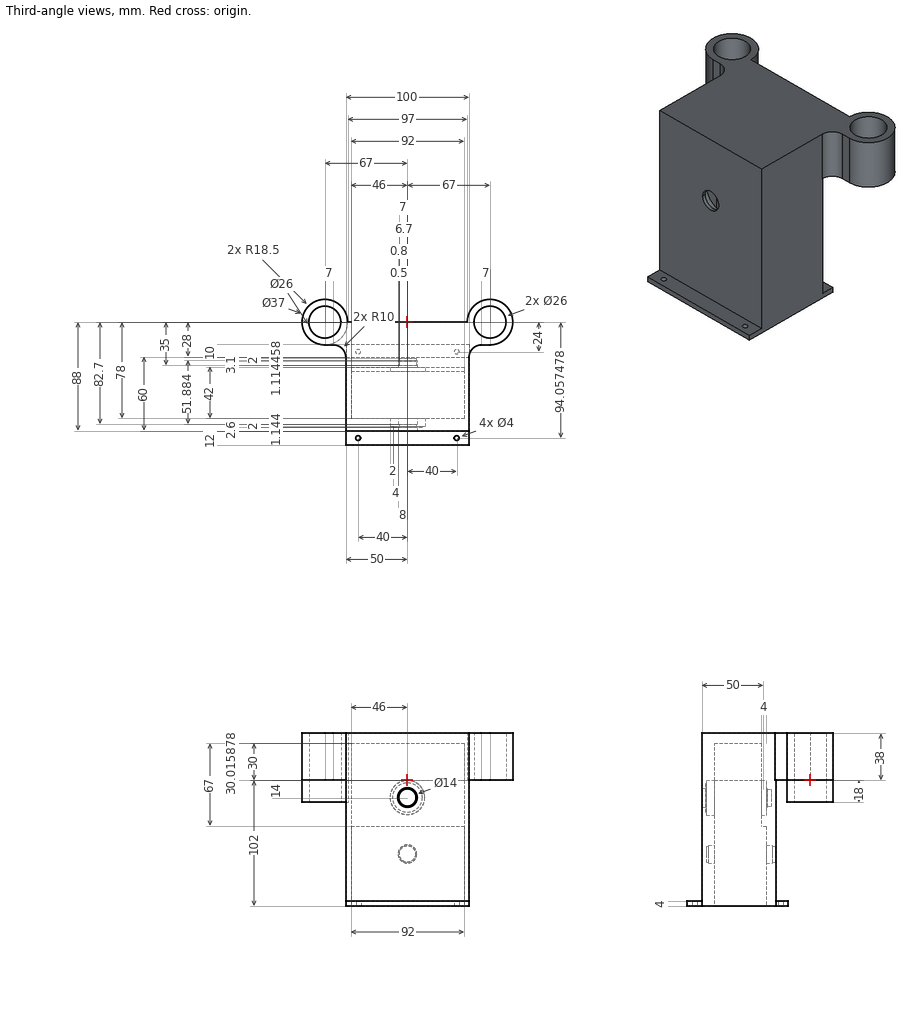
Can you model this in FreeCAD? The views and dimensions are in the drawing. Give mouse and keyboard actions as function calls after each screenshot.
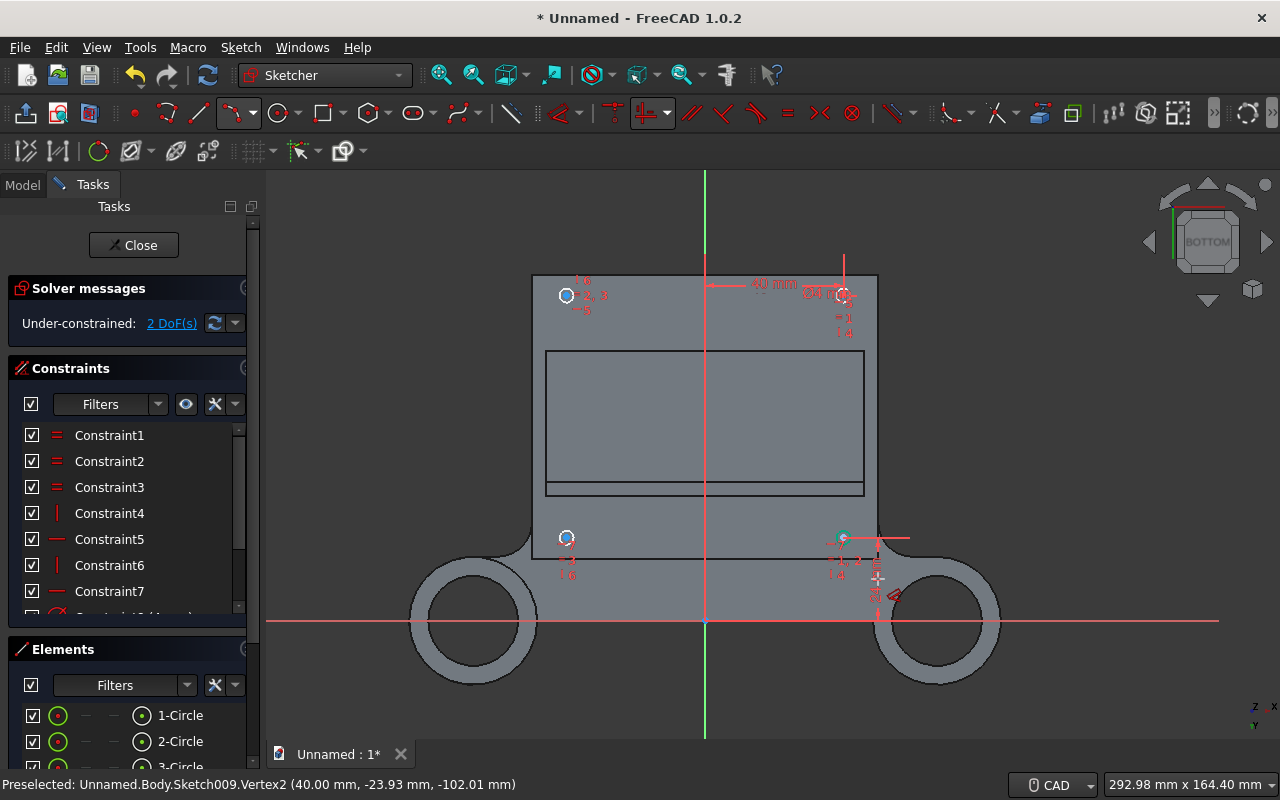
click(567, 296)
click(636, 655)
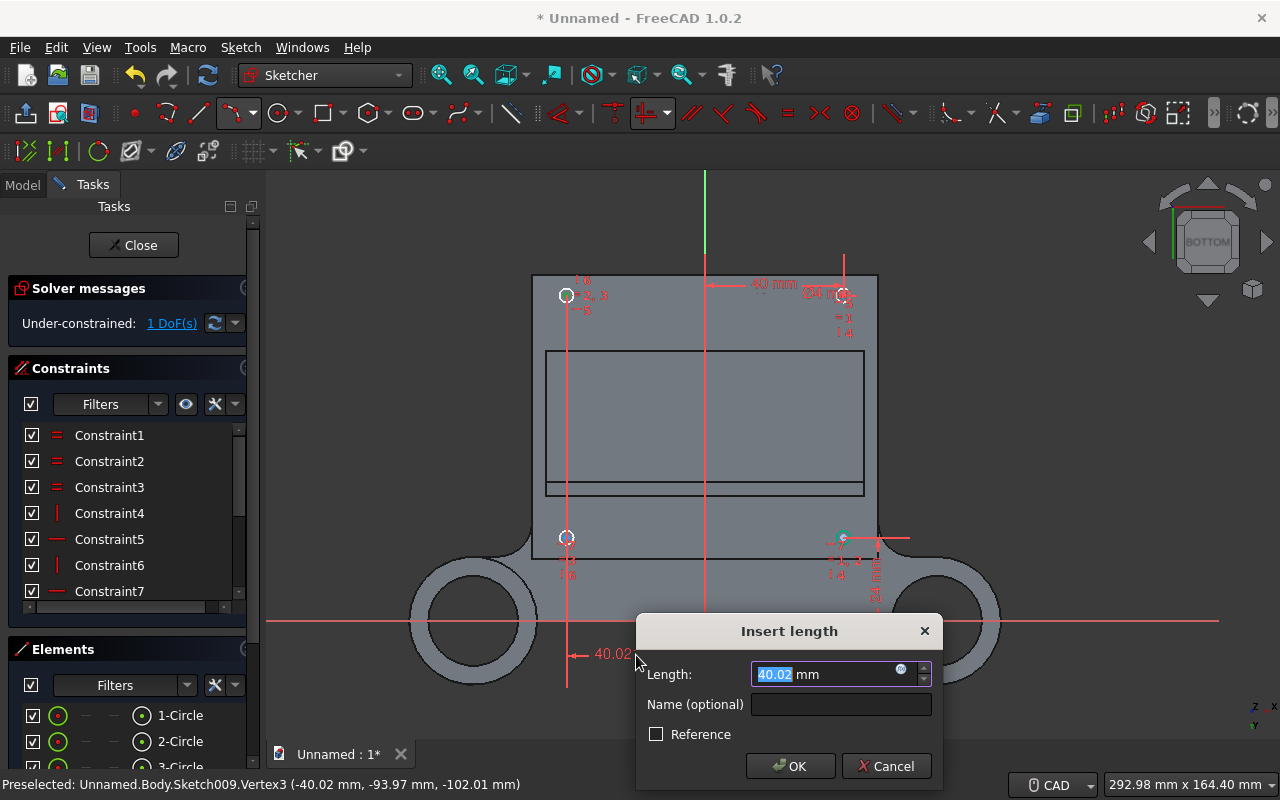
text(40)
key(Return)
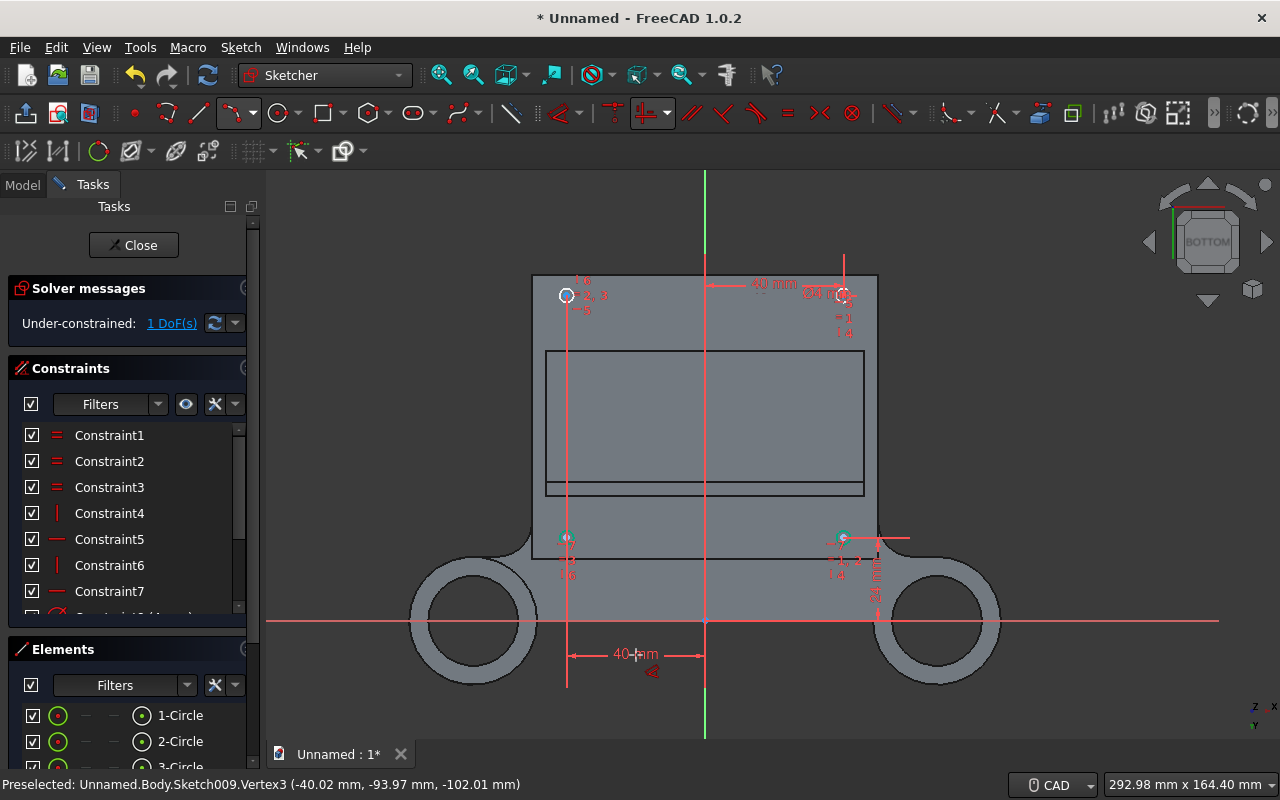
click(844, 296)
click(878, 458)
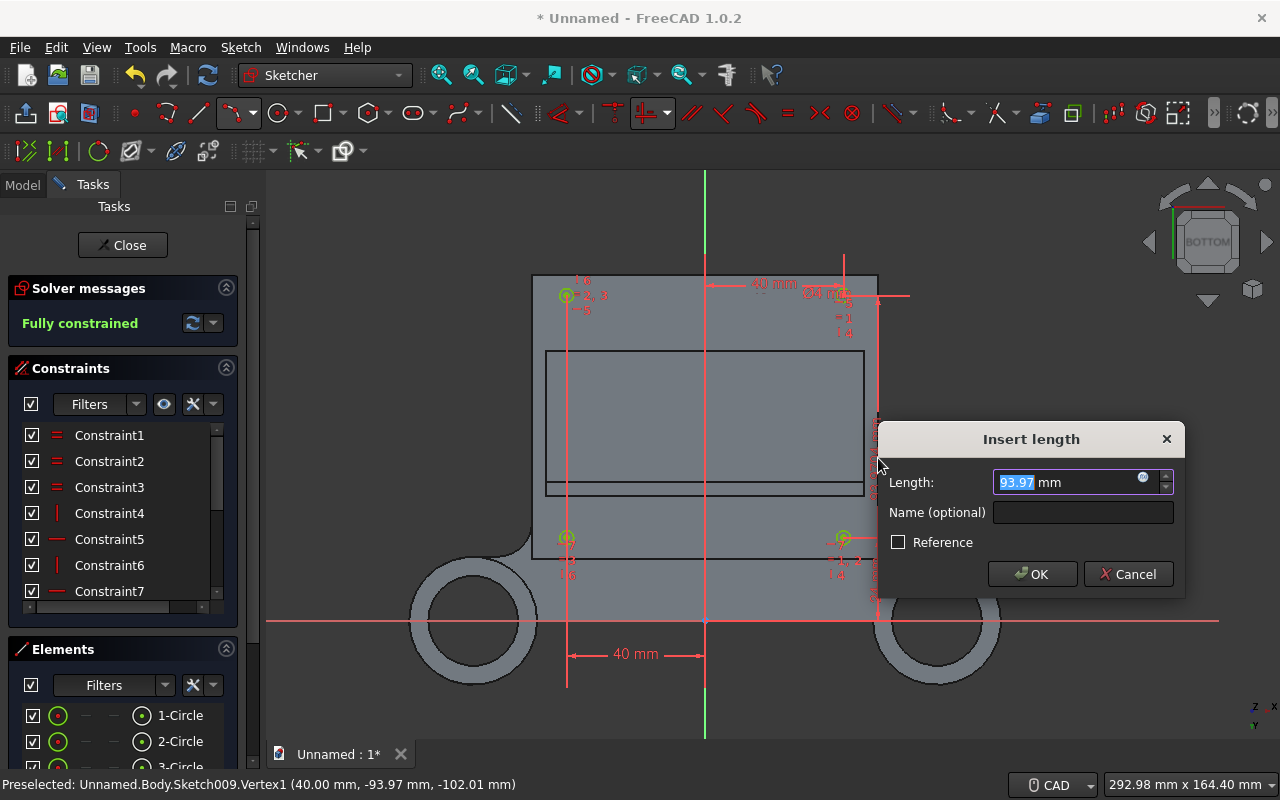
text(94.057478)
key(Return)
key(Escape)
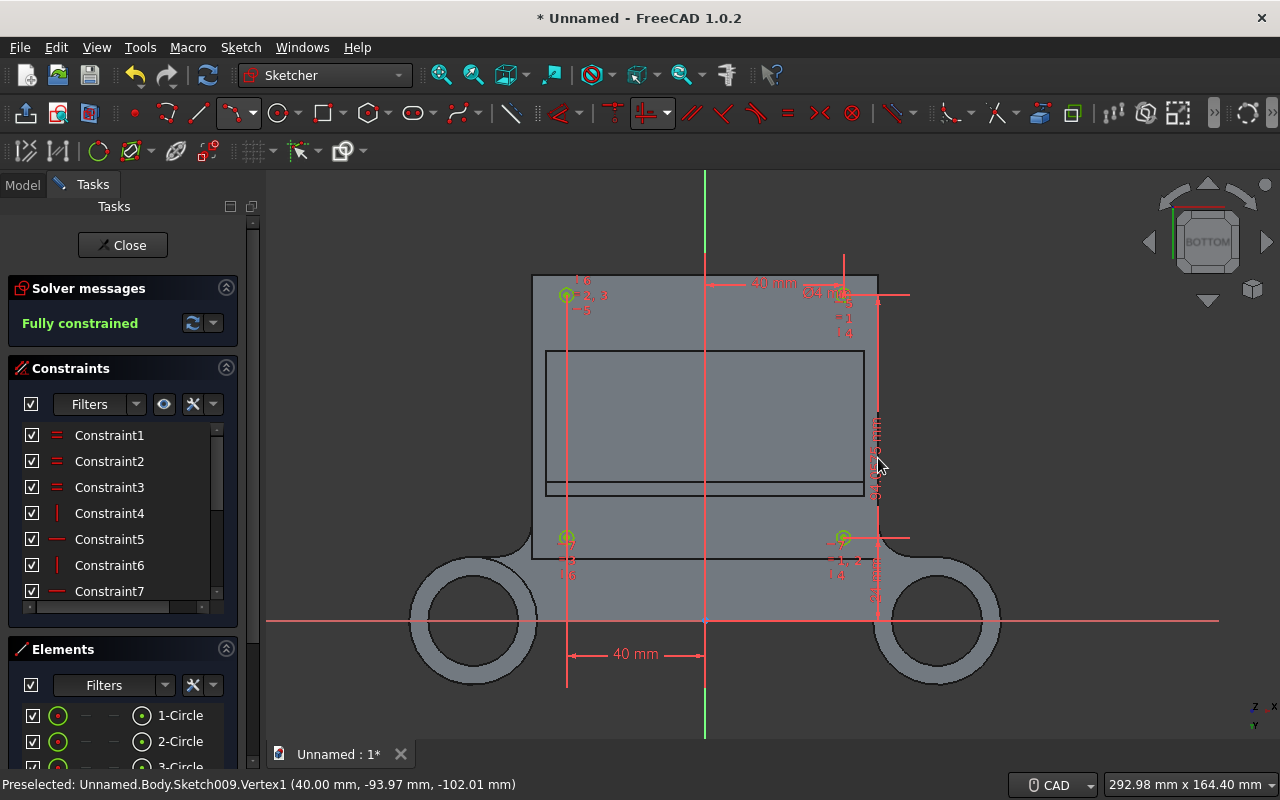
click(123, 245)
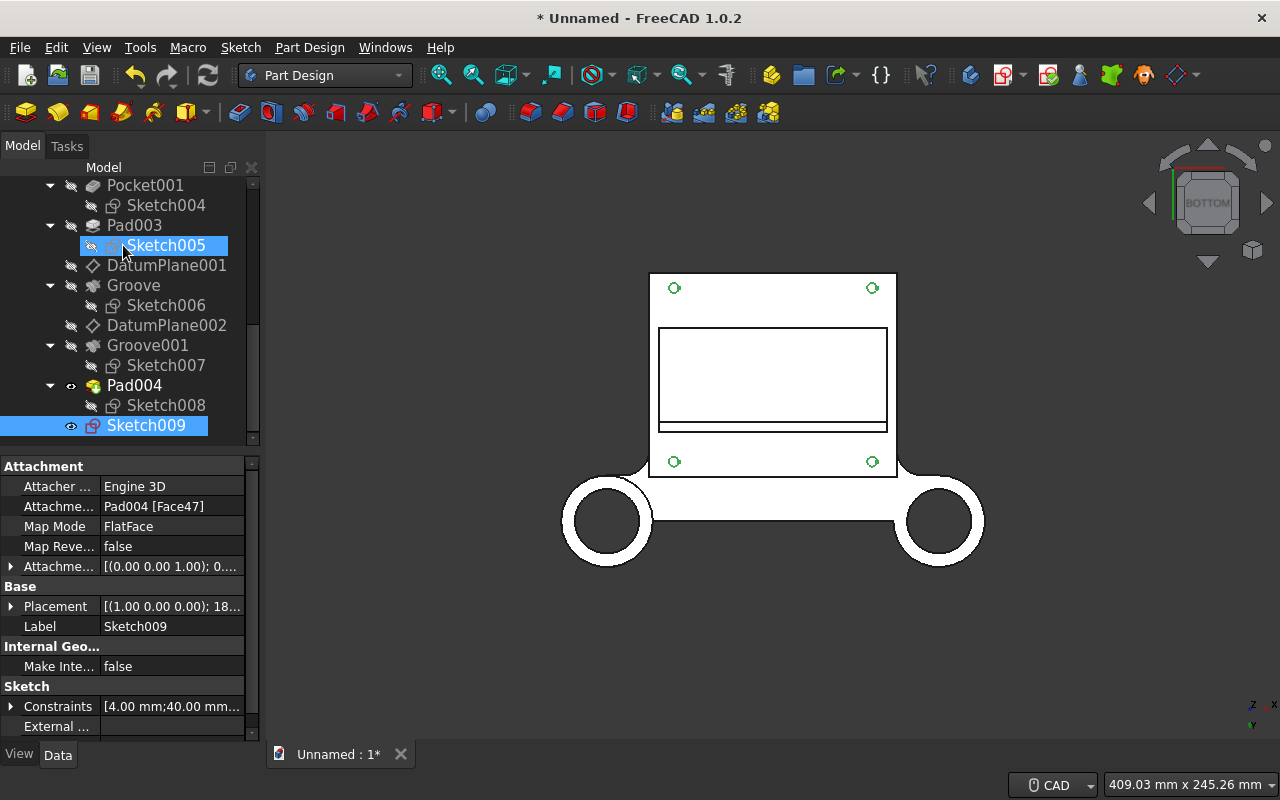
click(240, 112)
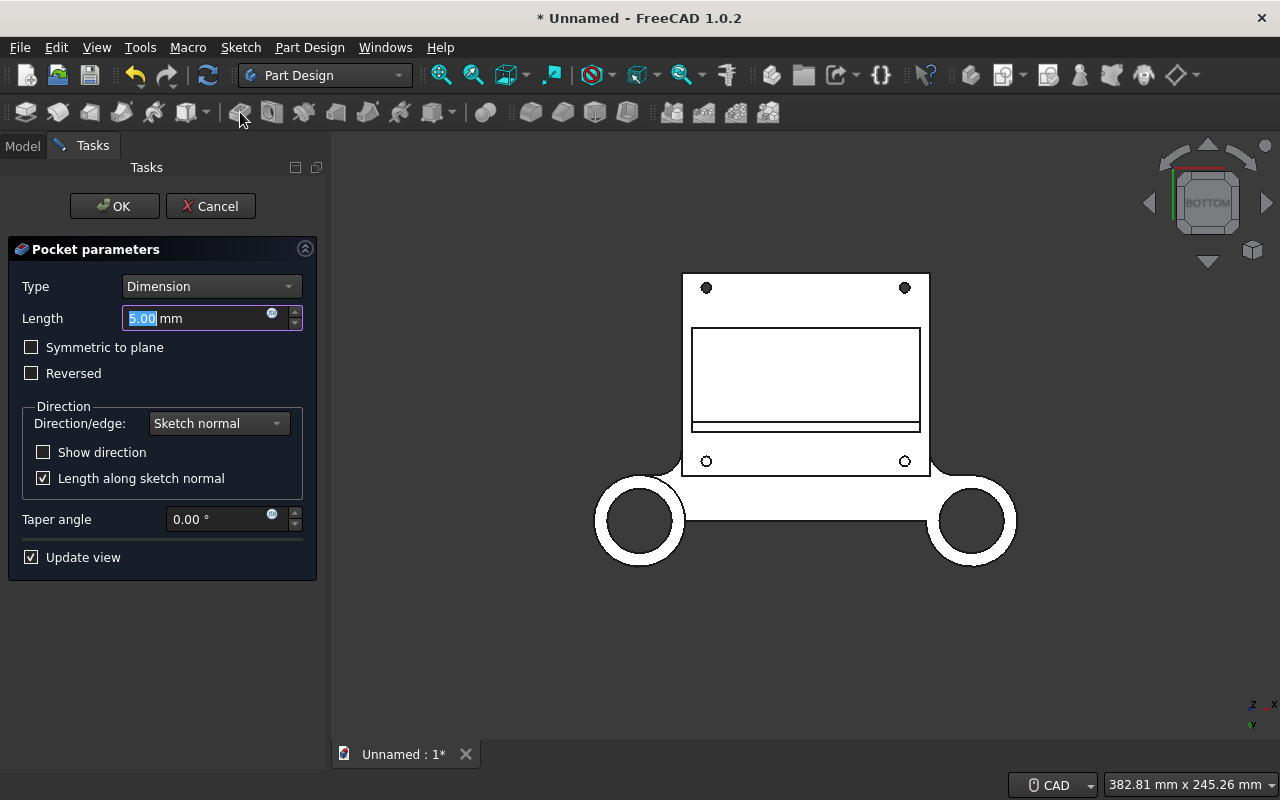
text(4)
key(Tab)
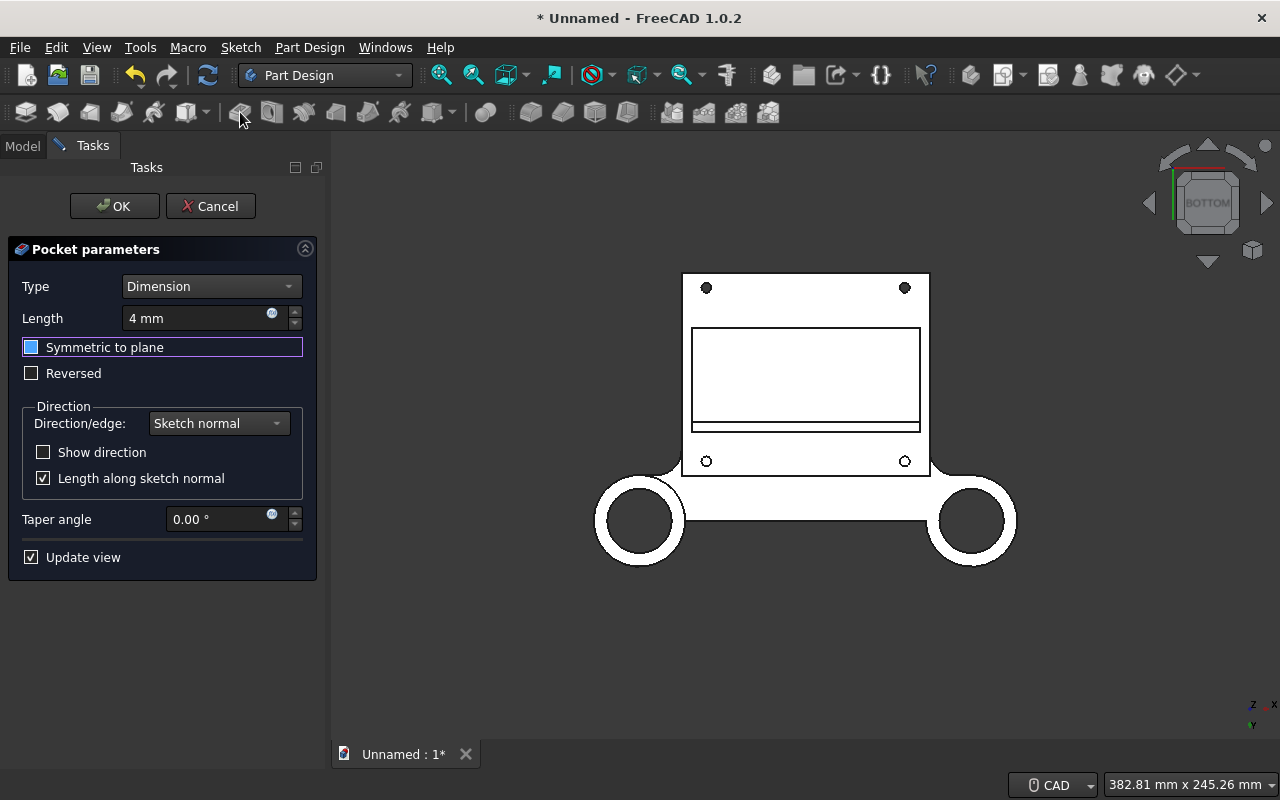
click(115, 206)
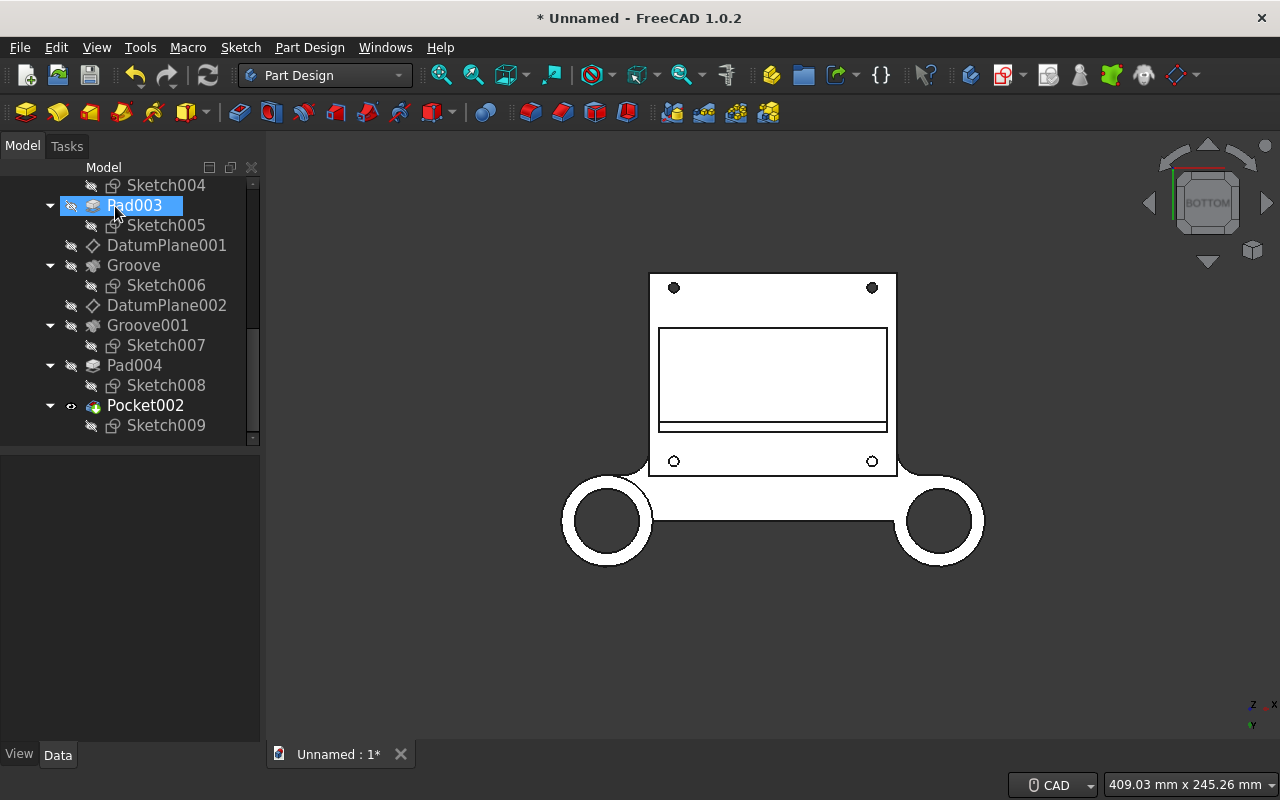
key(0)